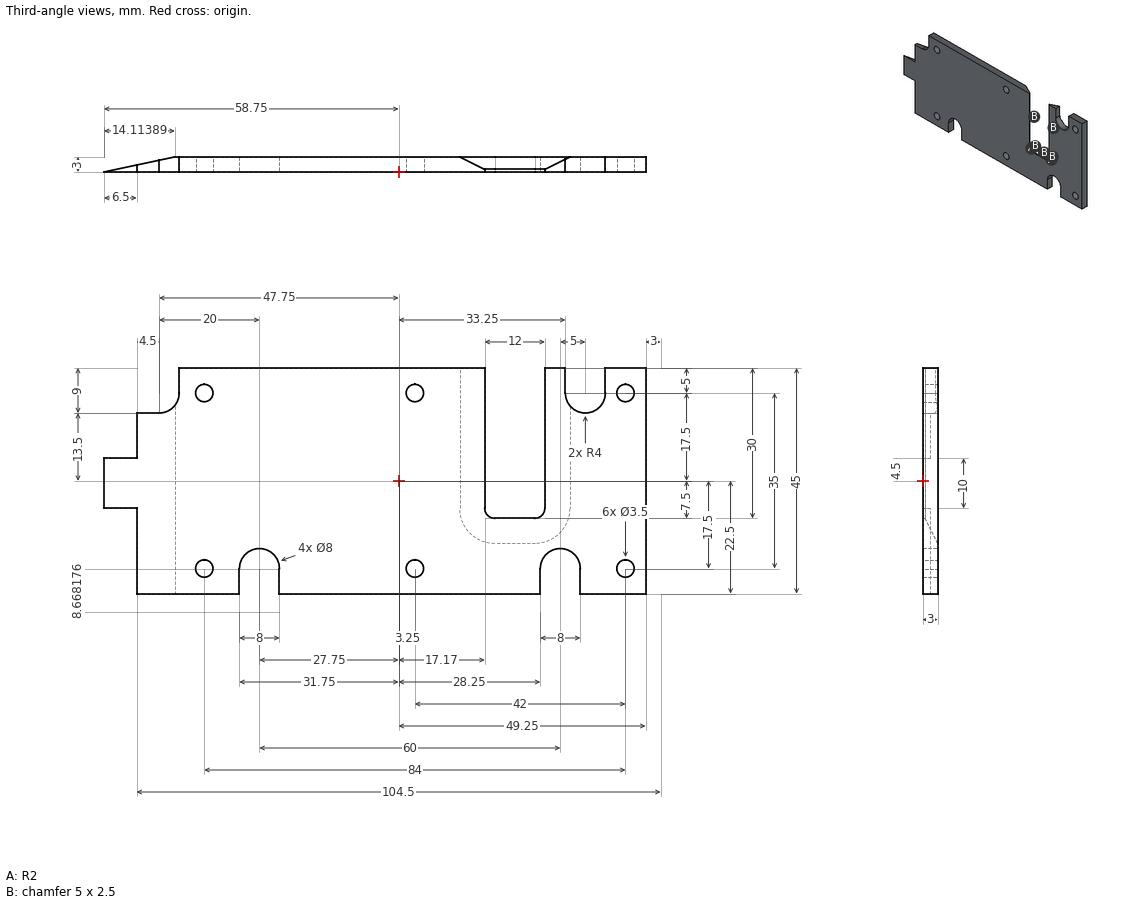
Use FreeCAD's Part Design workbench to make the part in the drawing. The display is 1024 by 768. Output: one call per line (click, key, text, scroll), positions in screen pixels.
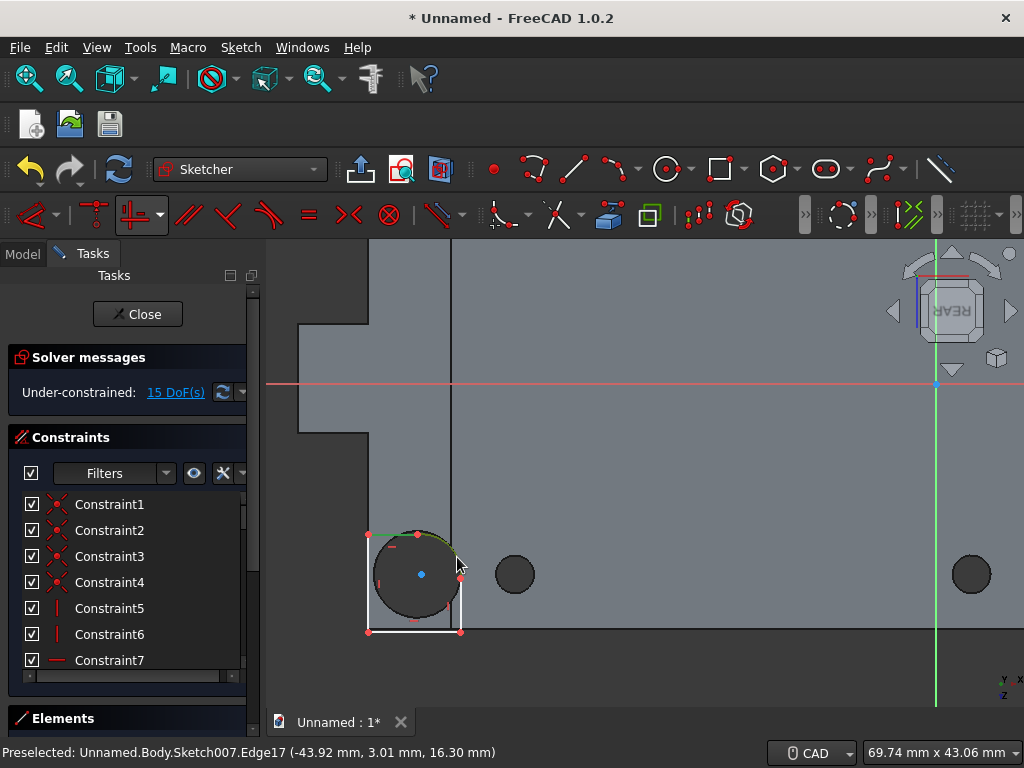
key(t)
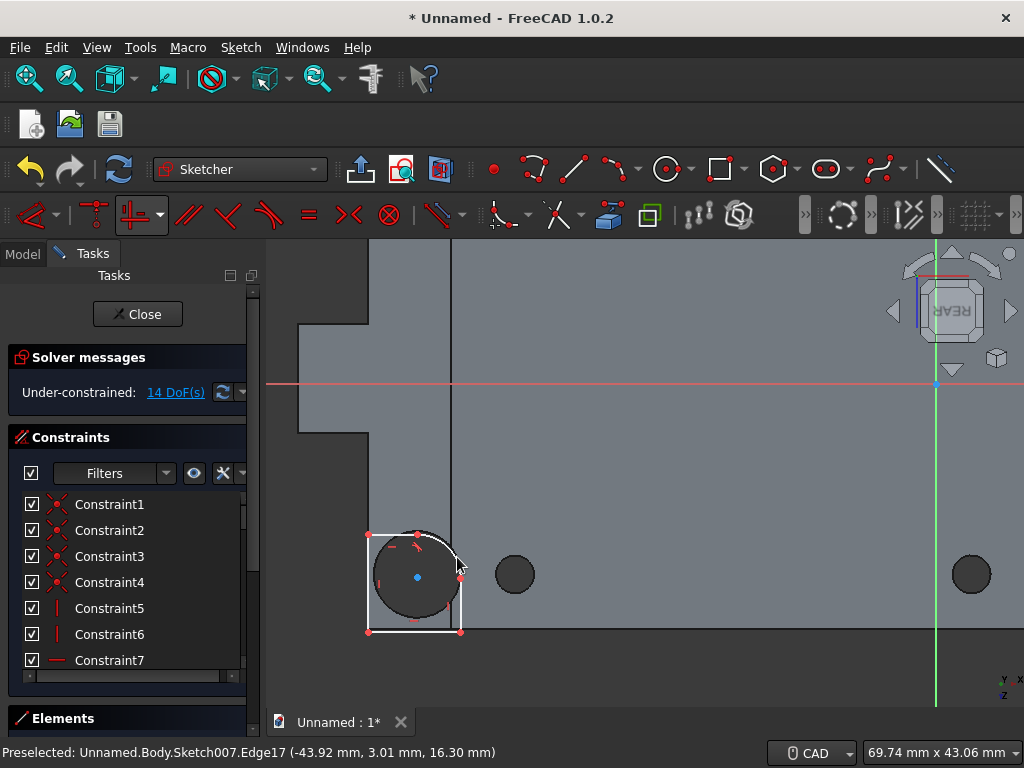
click(461, 616)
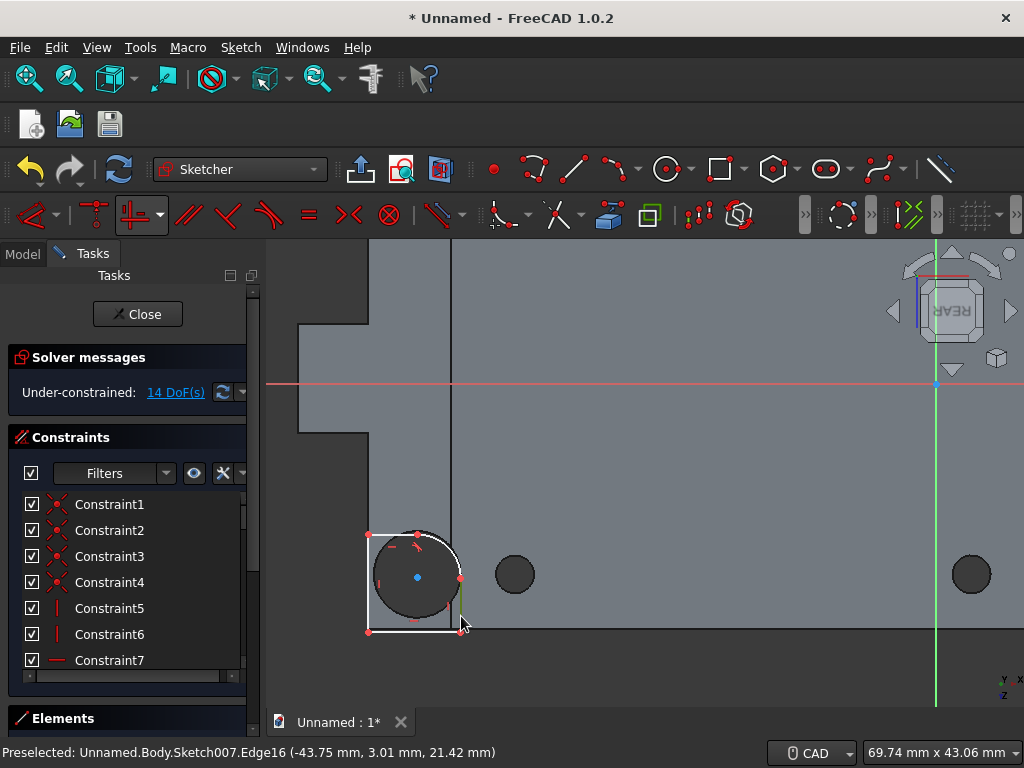
click(456, 558)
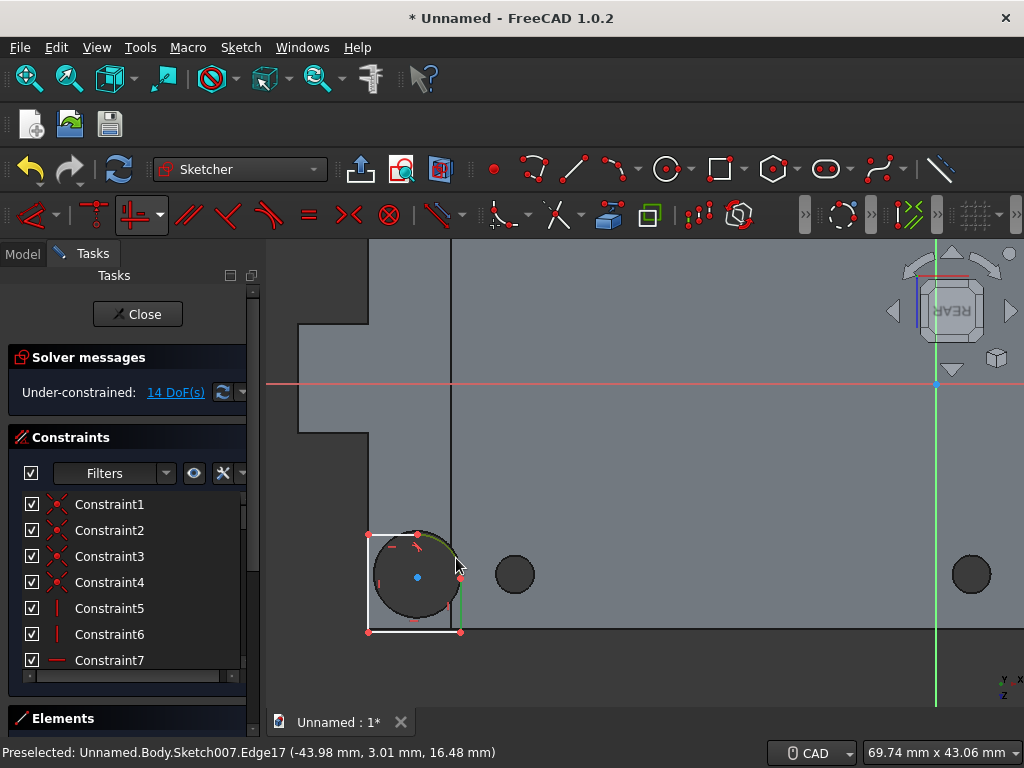
click(270, 216)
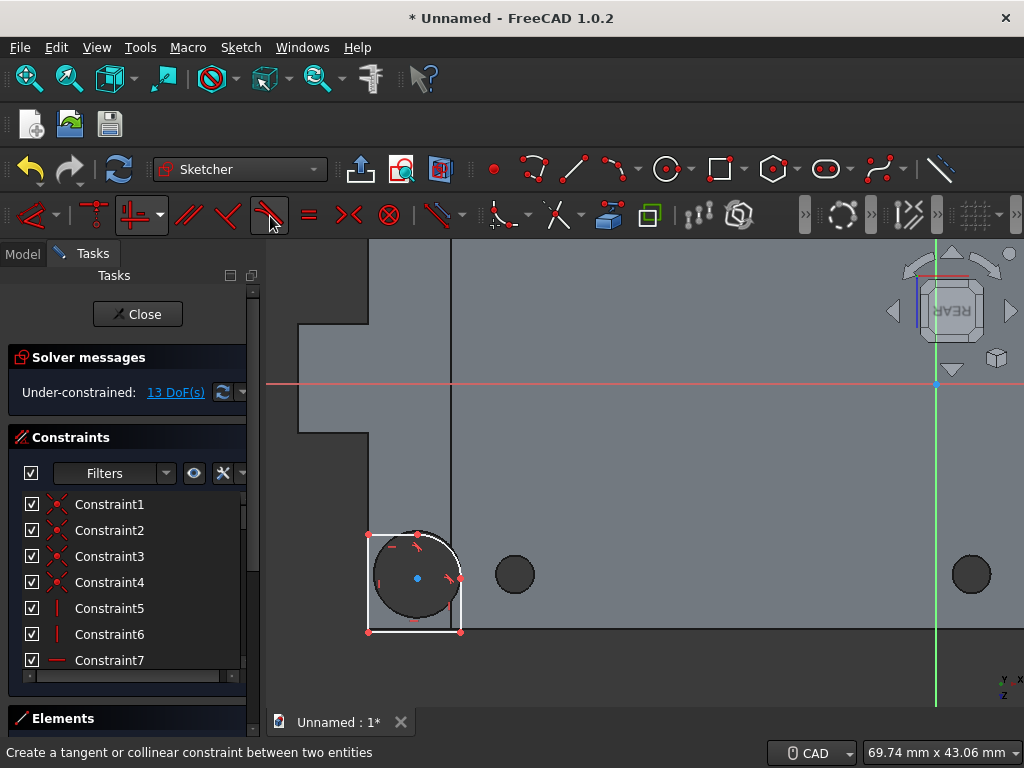
scroll(402, 536, down, 5)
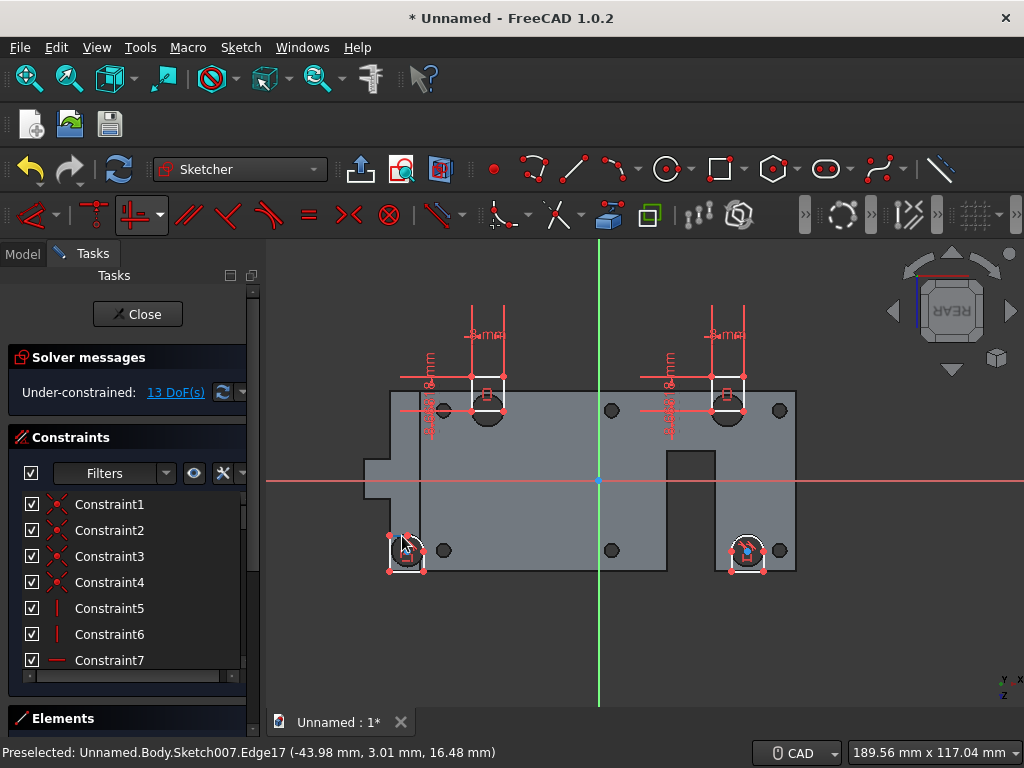
click(748, 536)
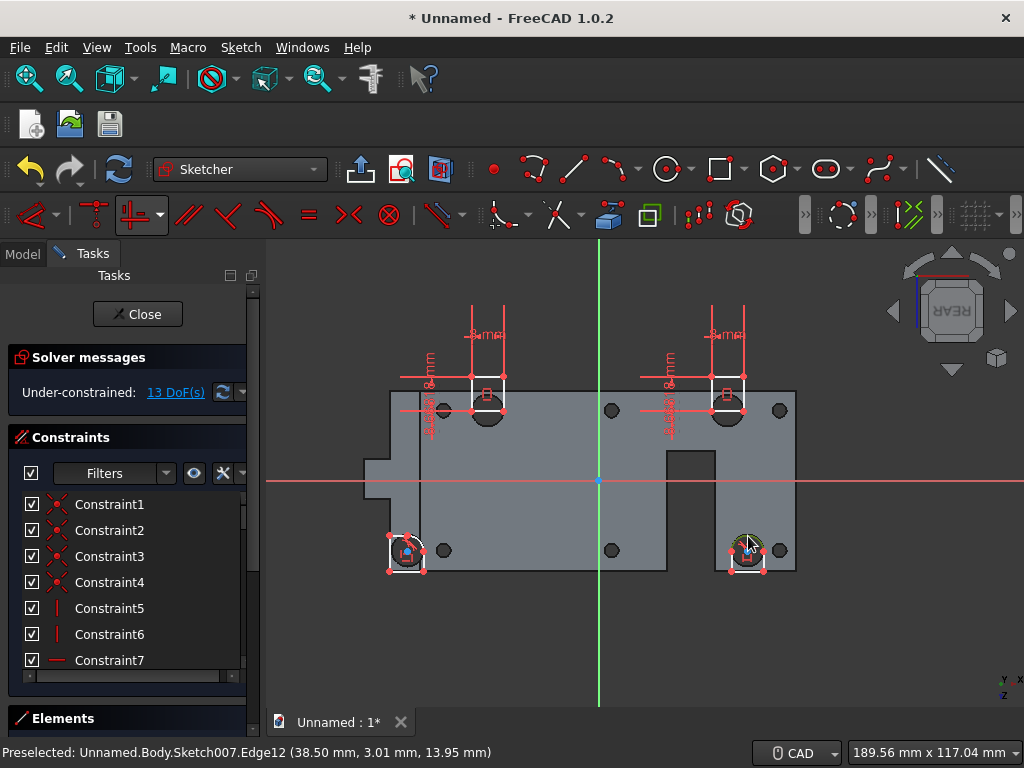
click(419, 541)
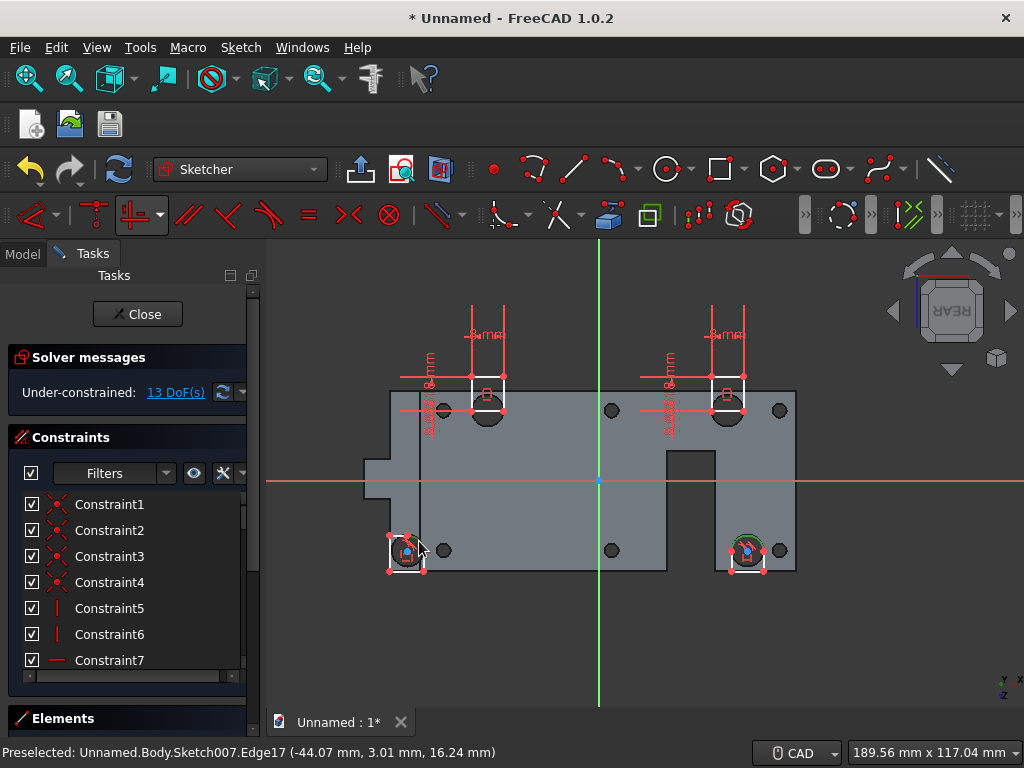
key(e)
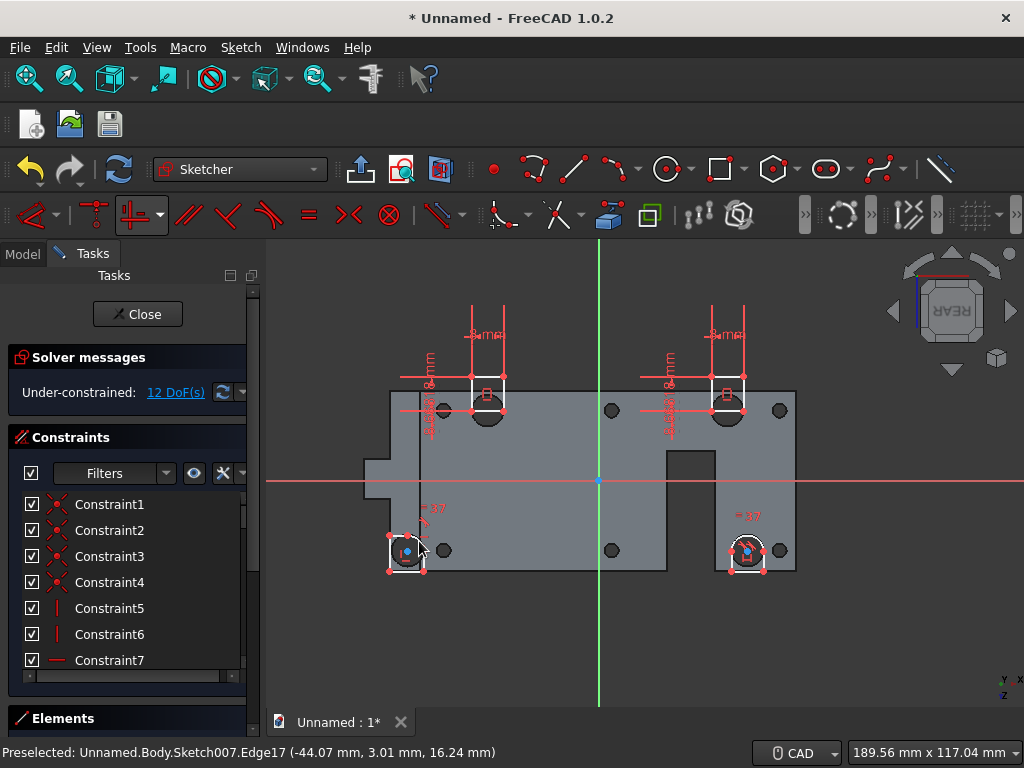
key(d)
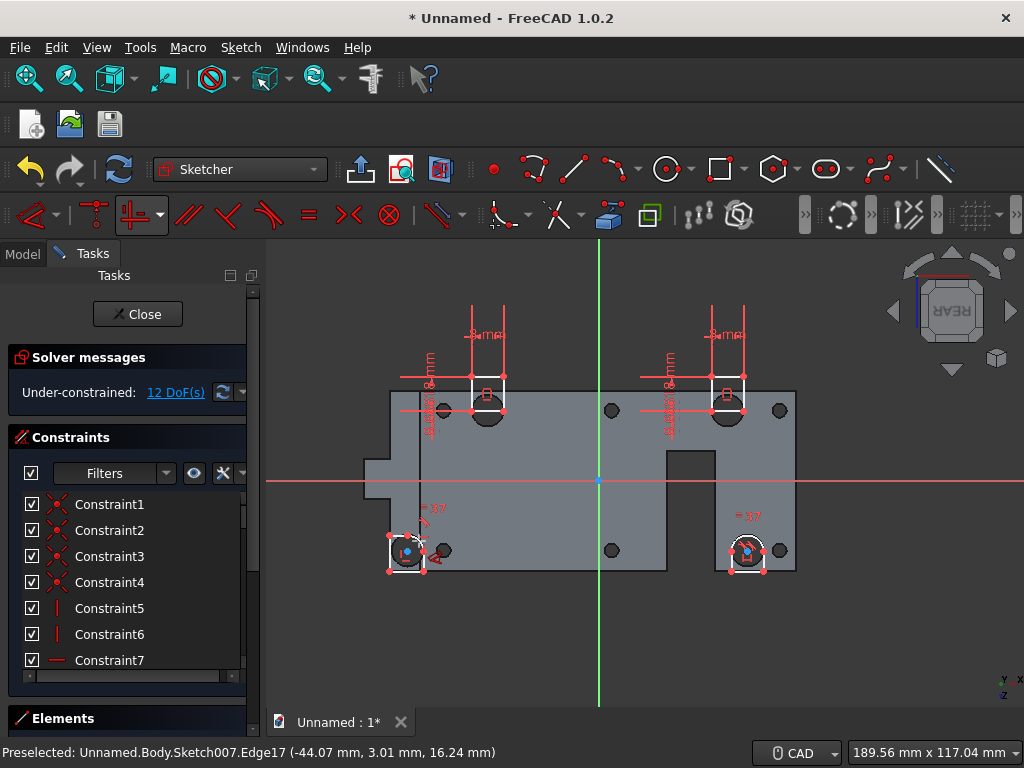
scroll(757, 539, up, 5)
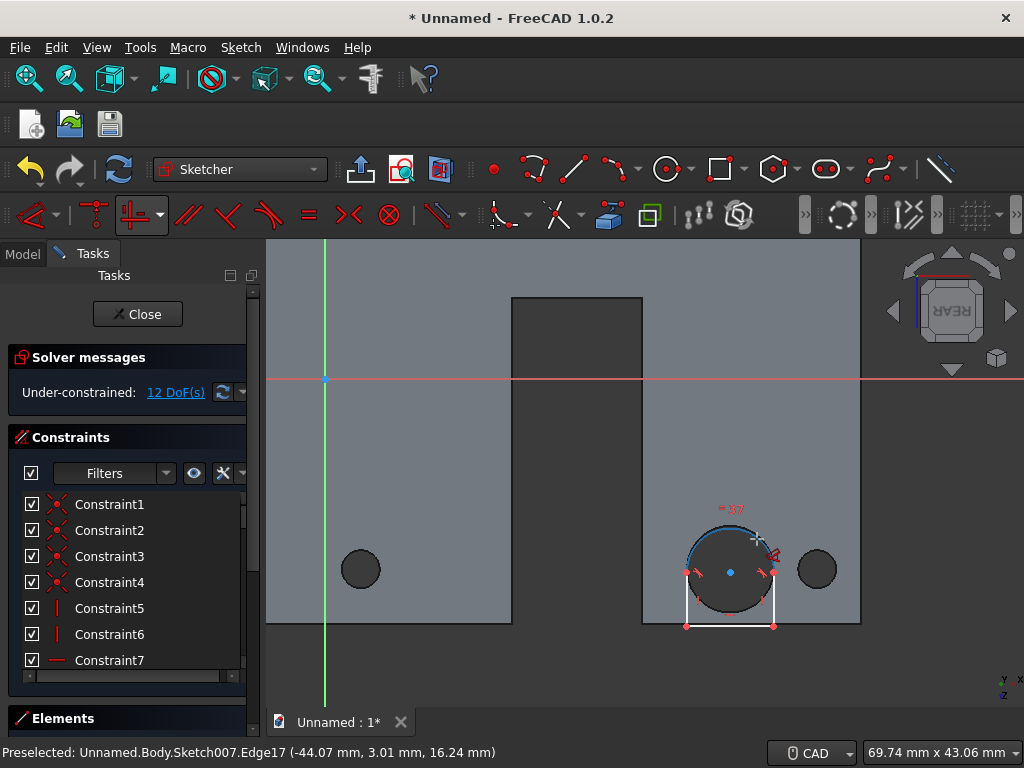
click(756, 537)
click(775, 511)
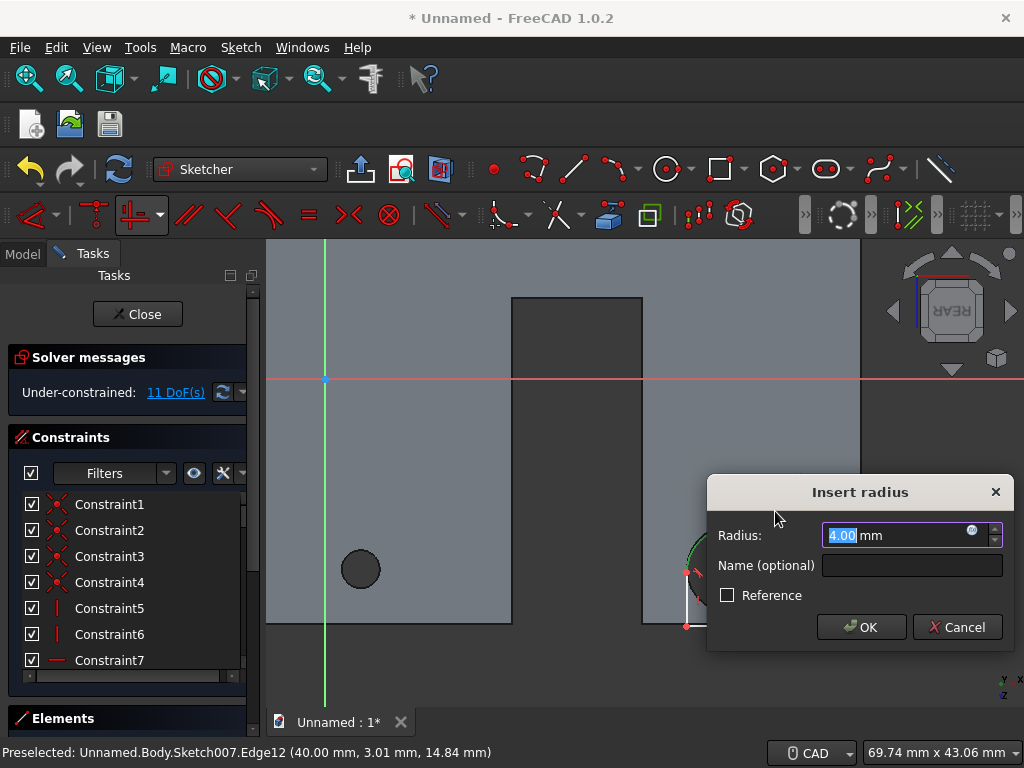
text(4)
key(Return)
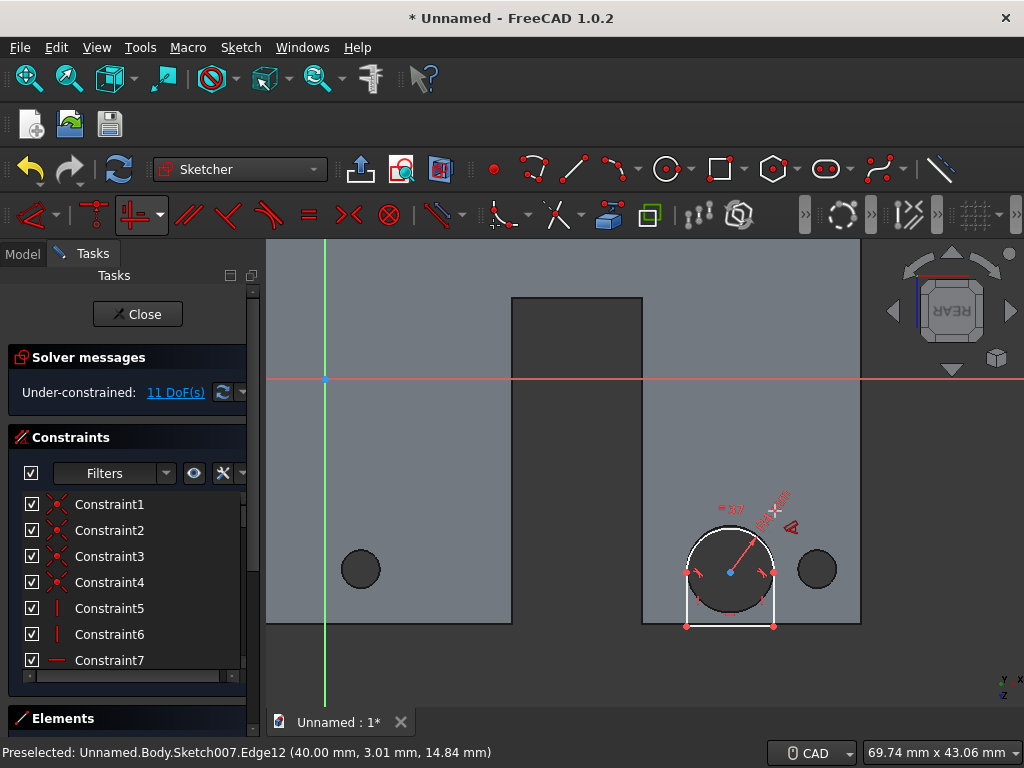
click(687, 588)
click(721, 599)